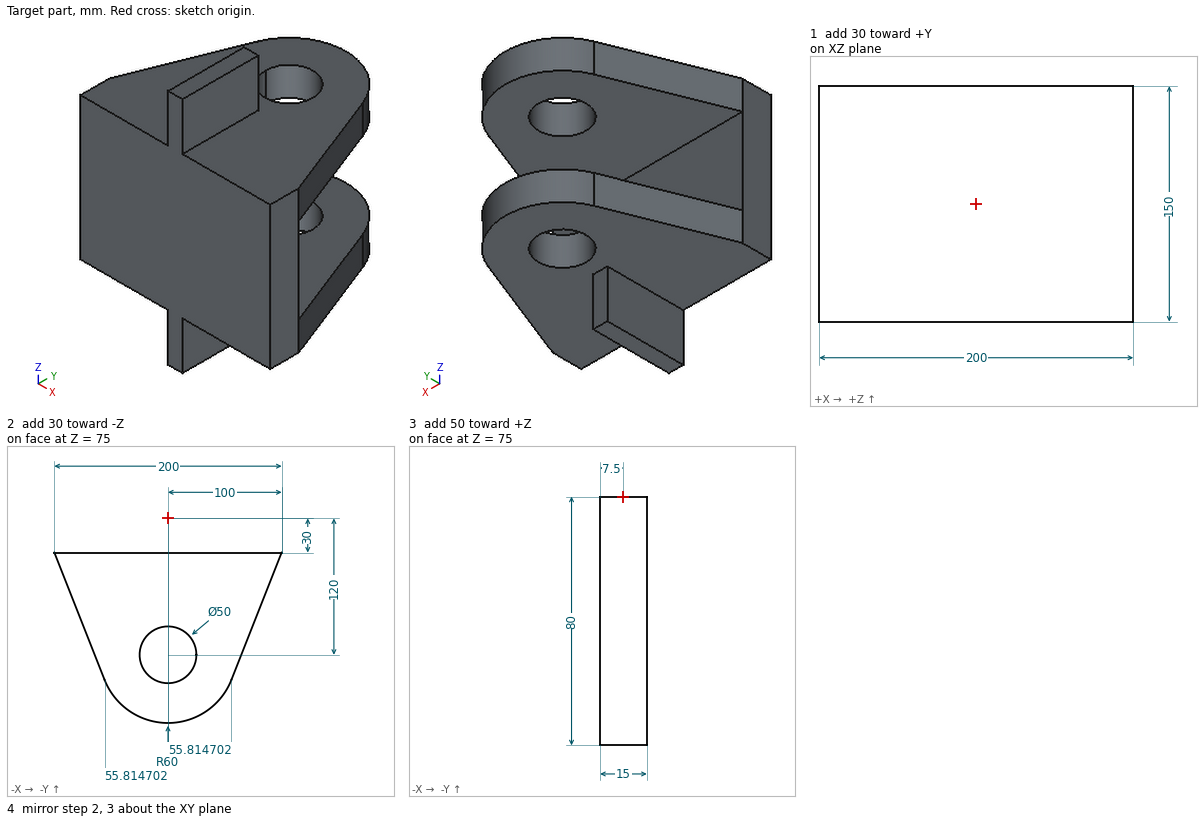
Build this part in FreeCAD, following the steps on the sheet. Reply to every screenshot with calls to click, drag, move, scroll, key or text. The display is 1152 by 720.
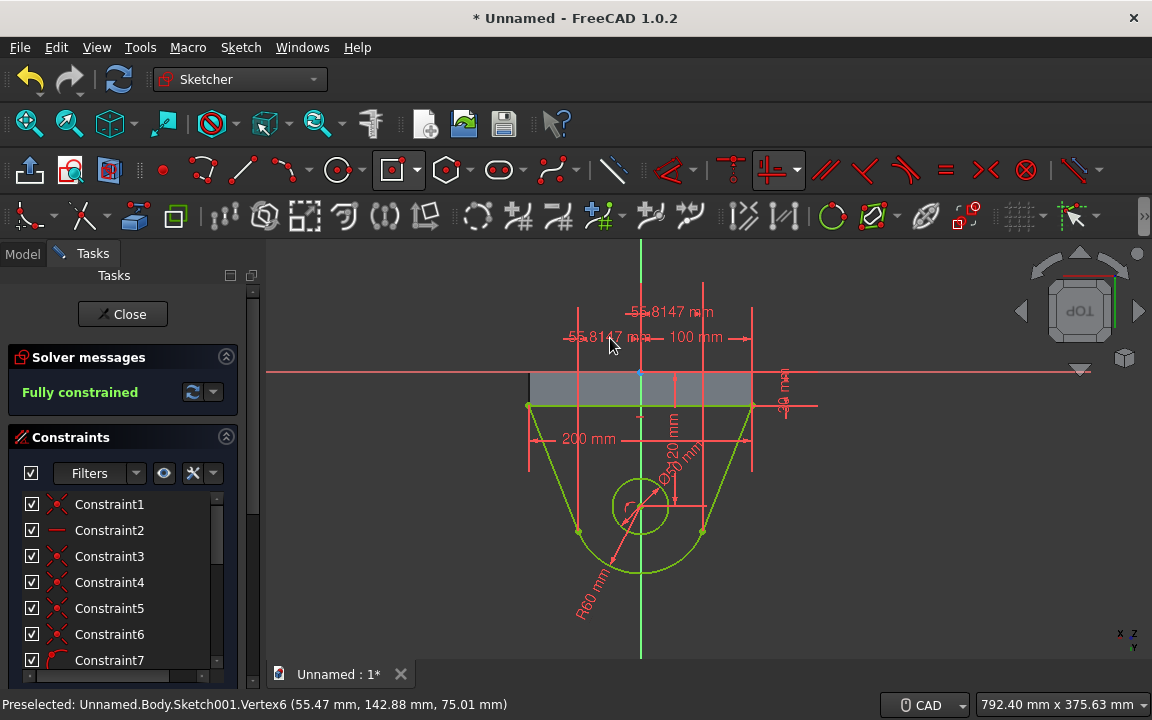
click(123, 314)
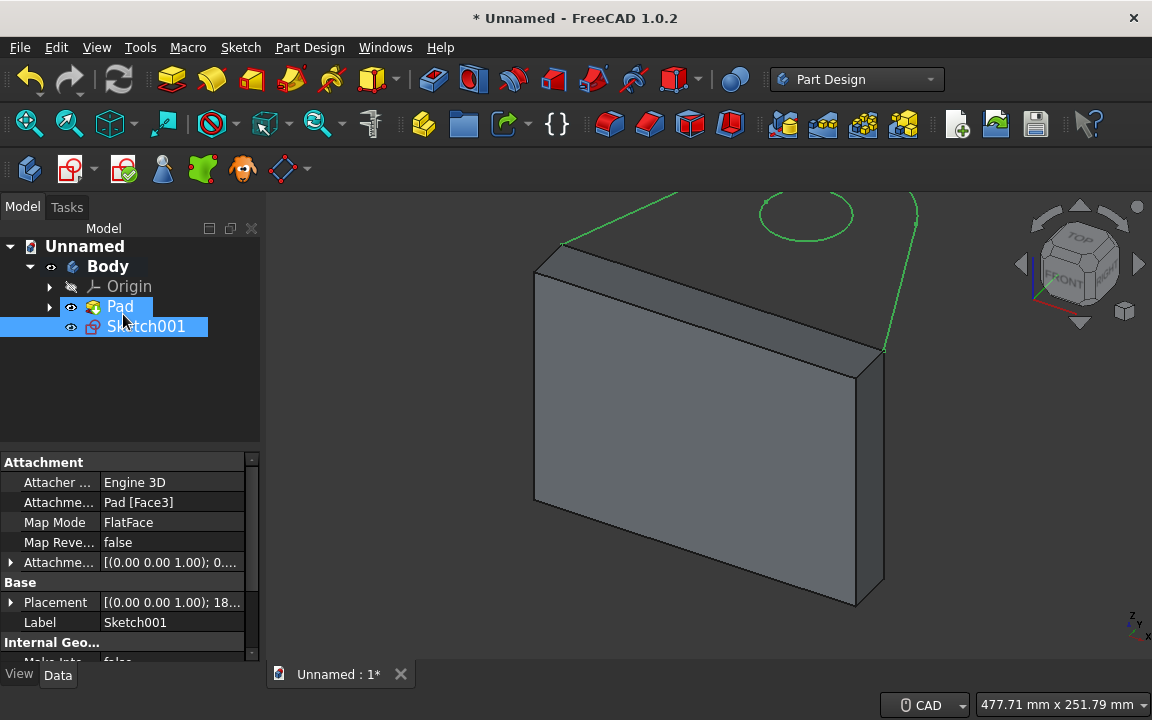
click(172, 80)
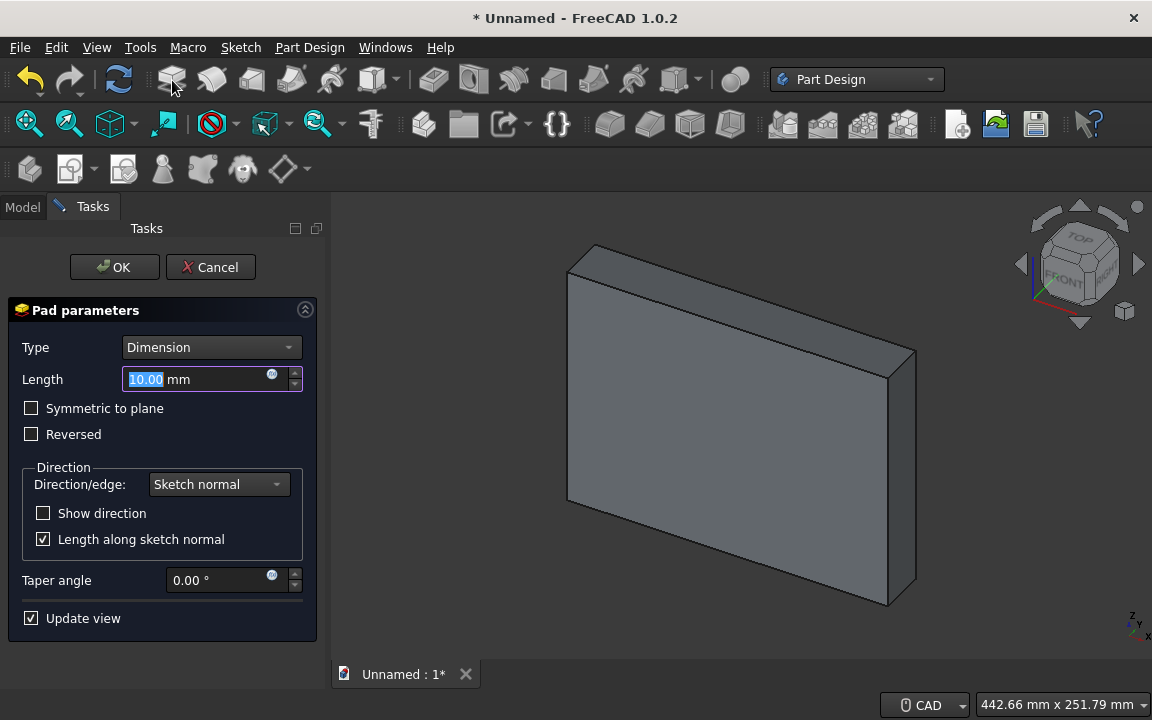
text(30)
key(Tab)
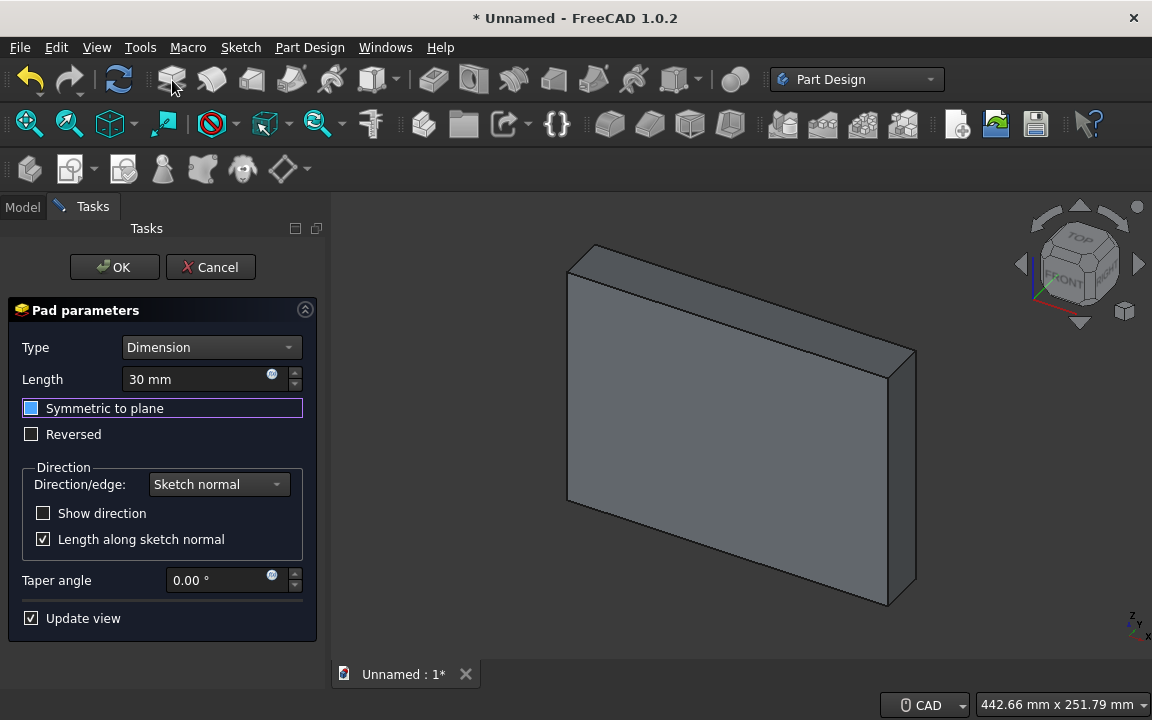
click(30, 434)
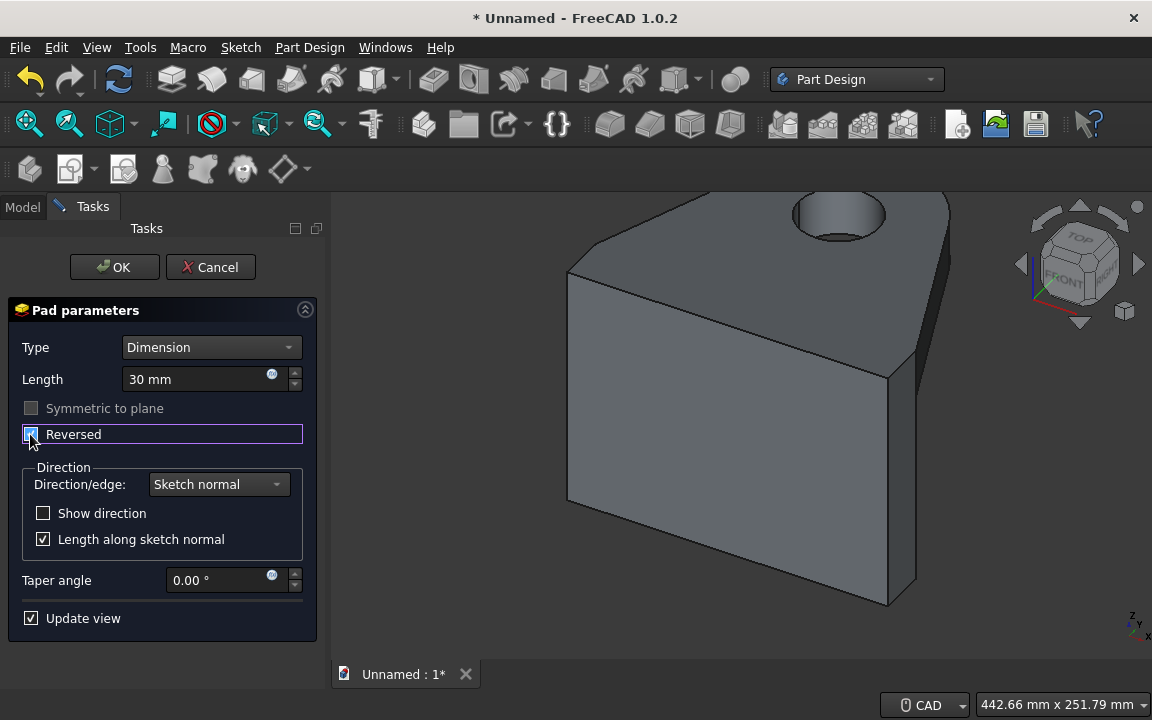
click(115, 267)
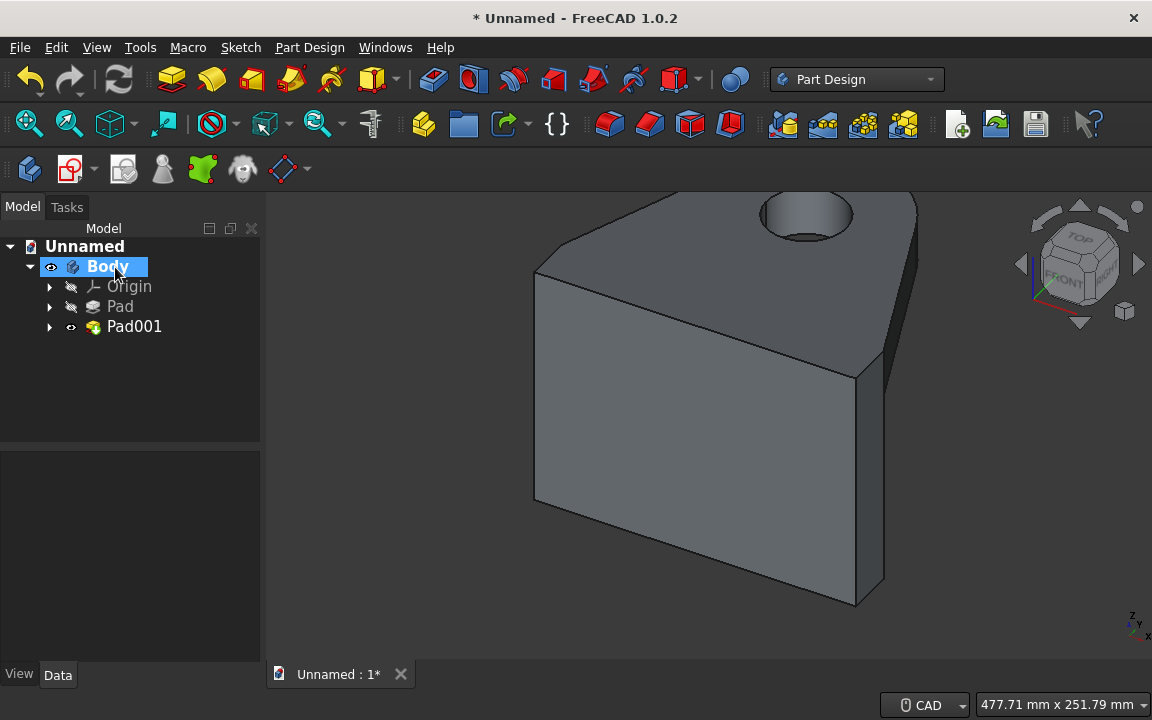
key(v)
key(f)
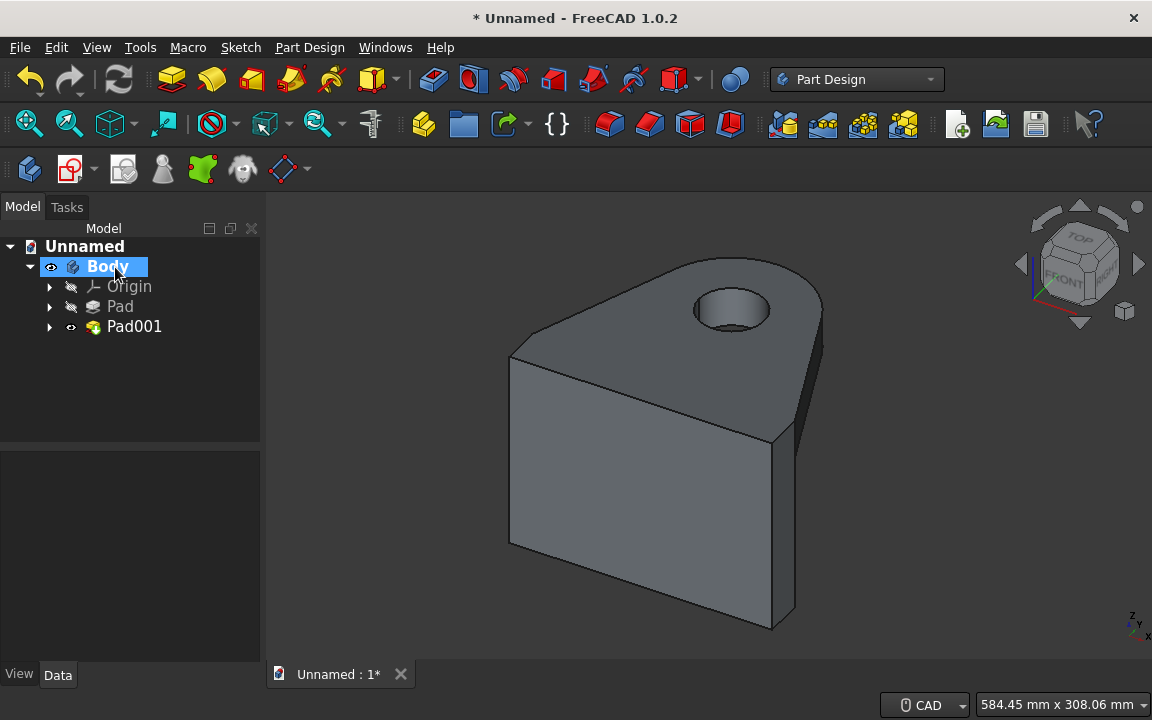
click(708, 383)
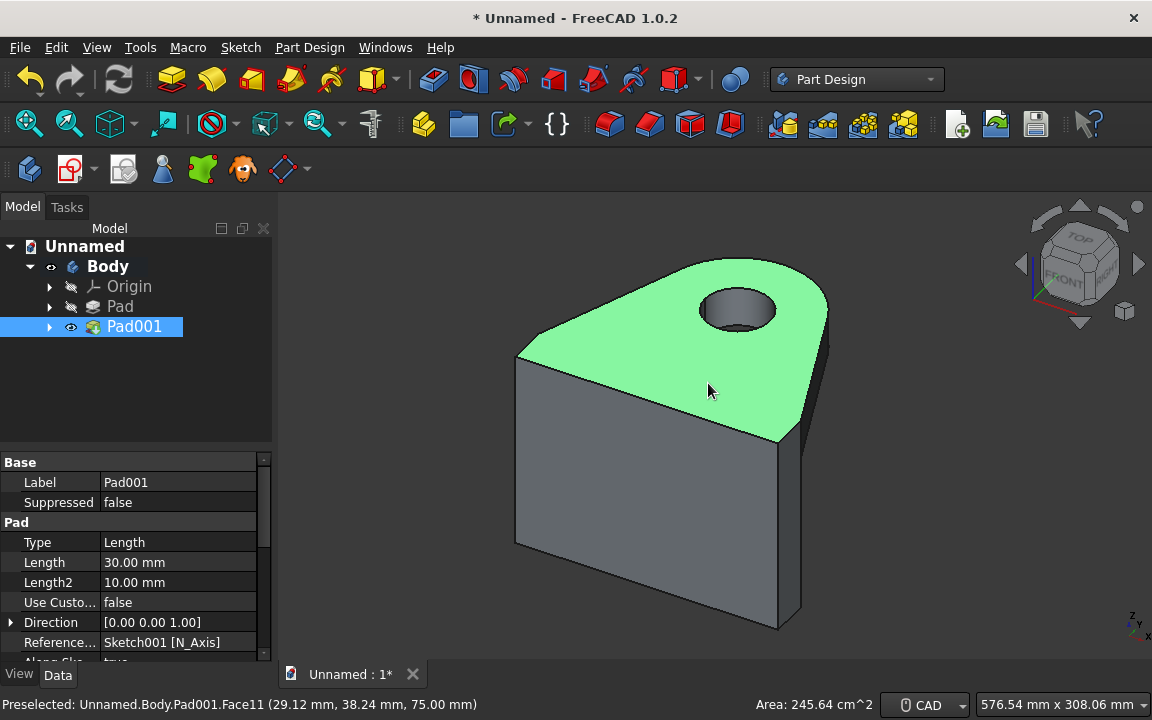
click(70, 170)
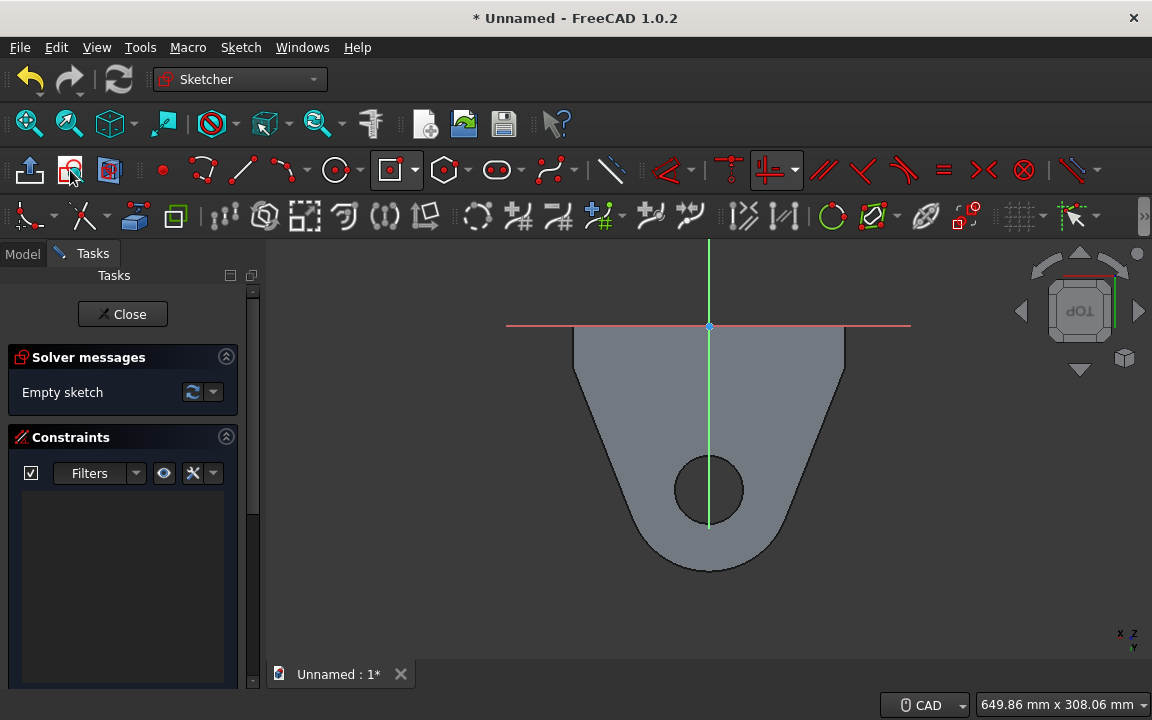
scroll(765, 325, up, 4)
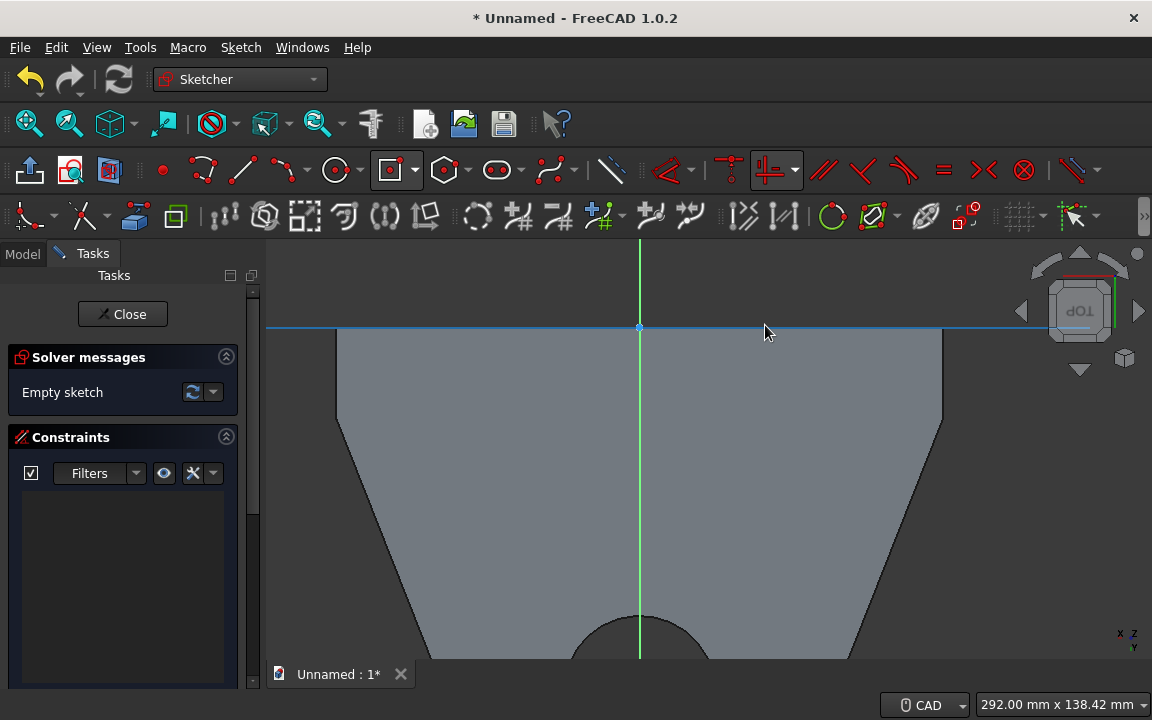
key(g)
key(r)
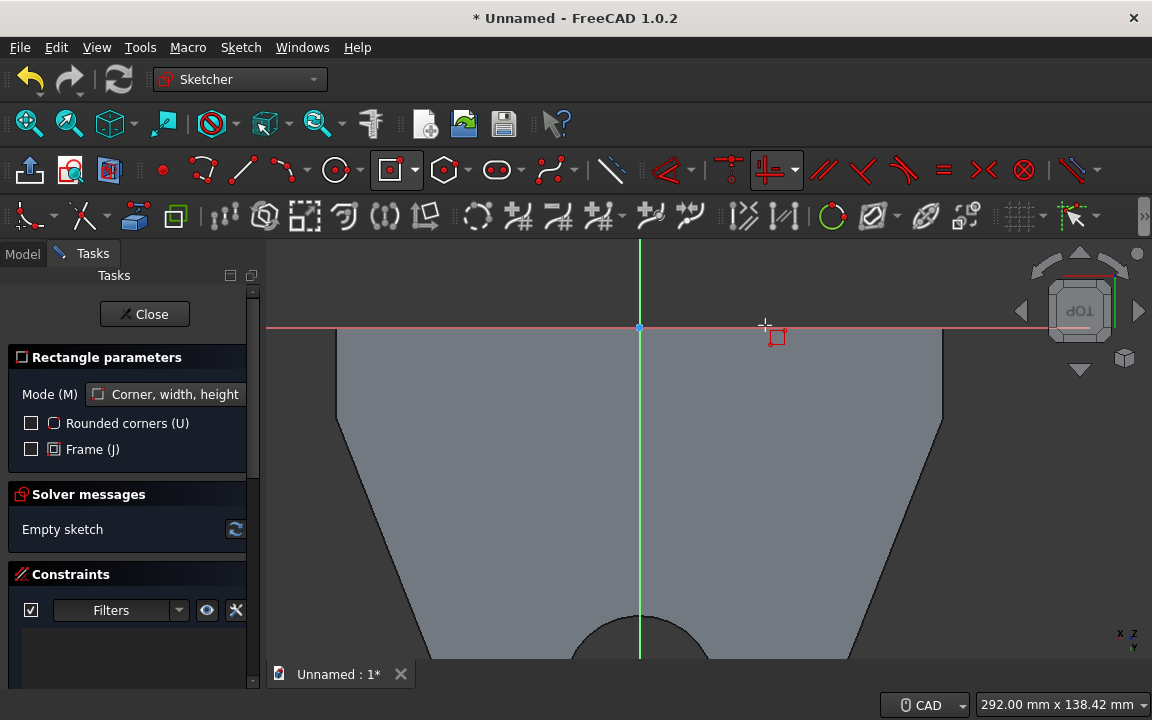
click(617, 328)
click(662, 570)
key(Escape)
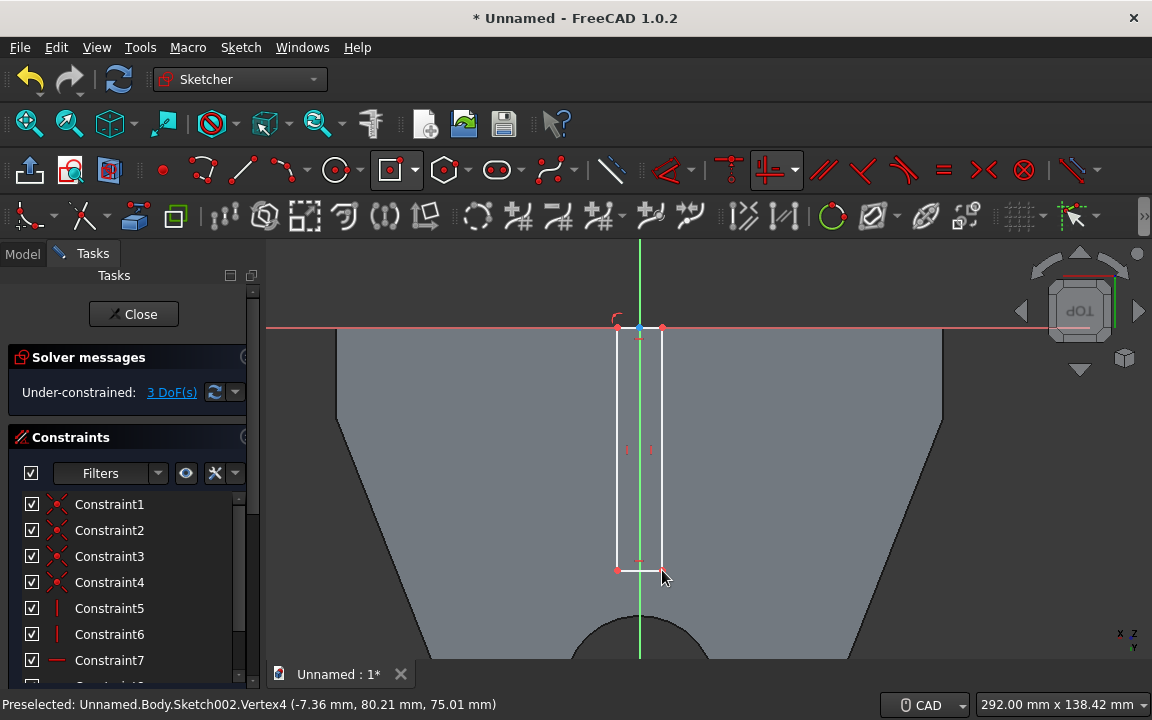
key(d)